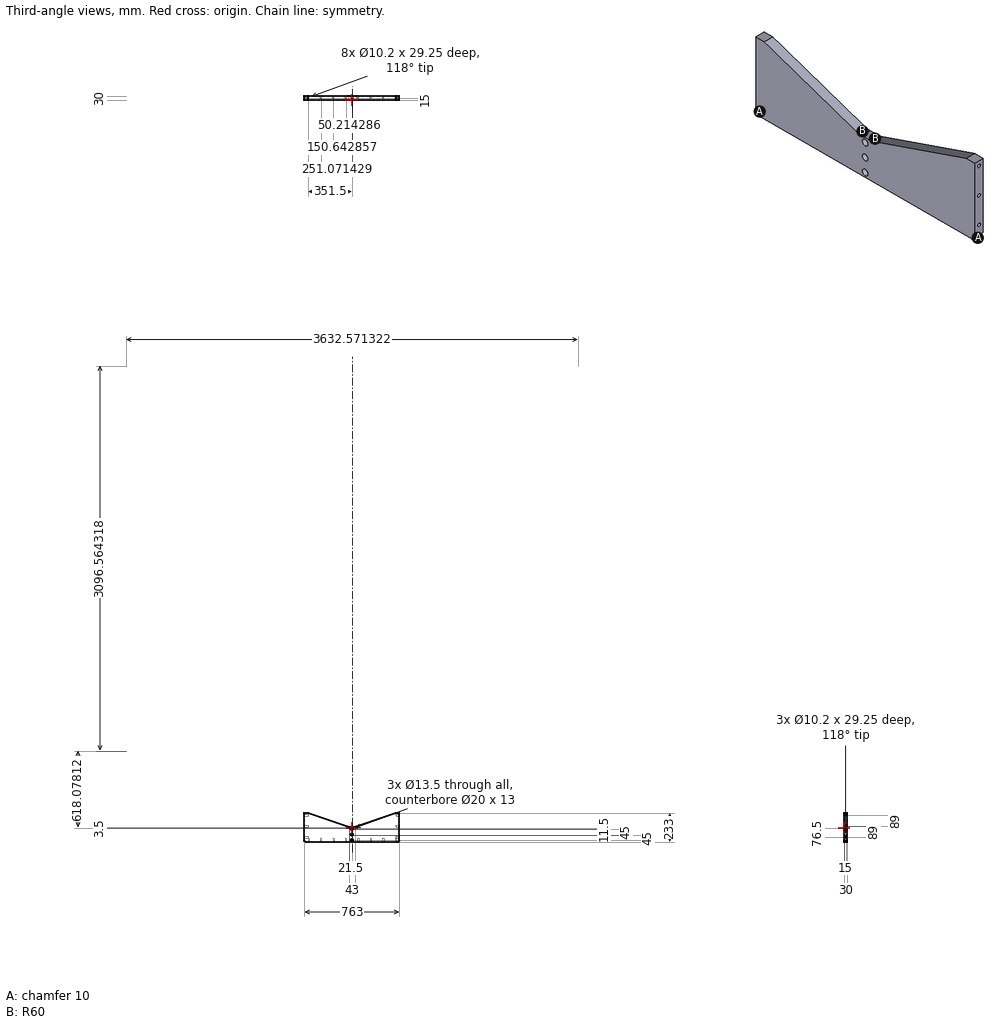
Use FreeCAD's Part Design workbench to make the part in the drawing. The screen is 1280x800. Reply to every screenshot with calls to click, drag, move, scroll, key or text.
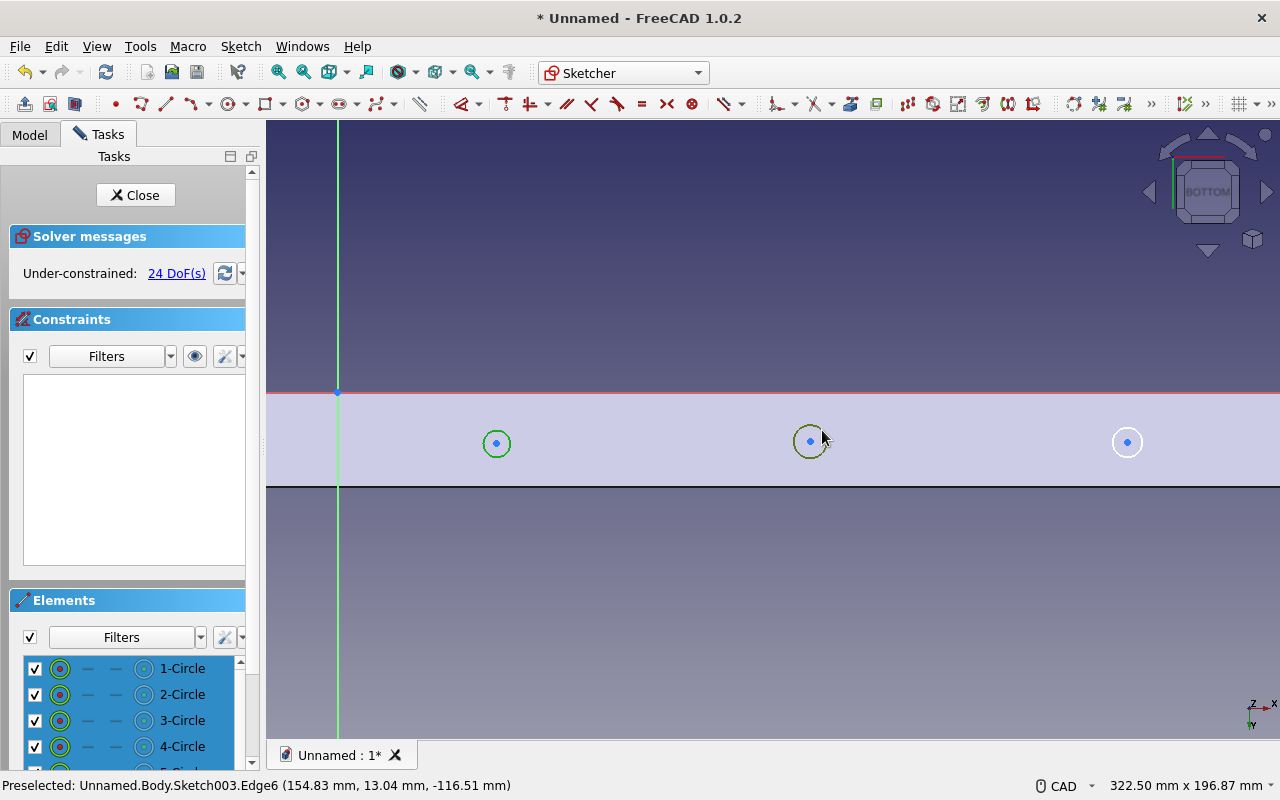
click(1113, 442)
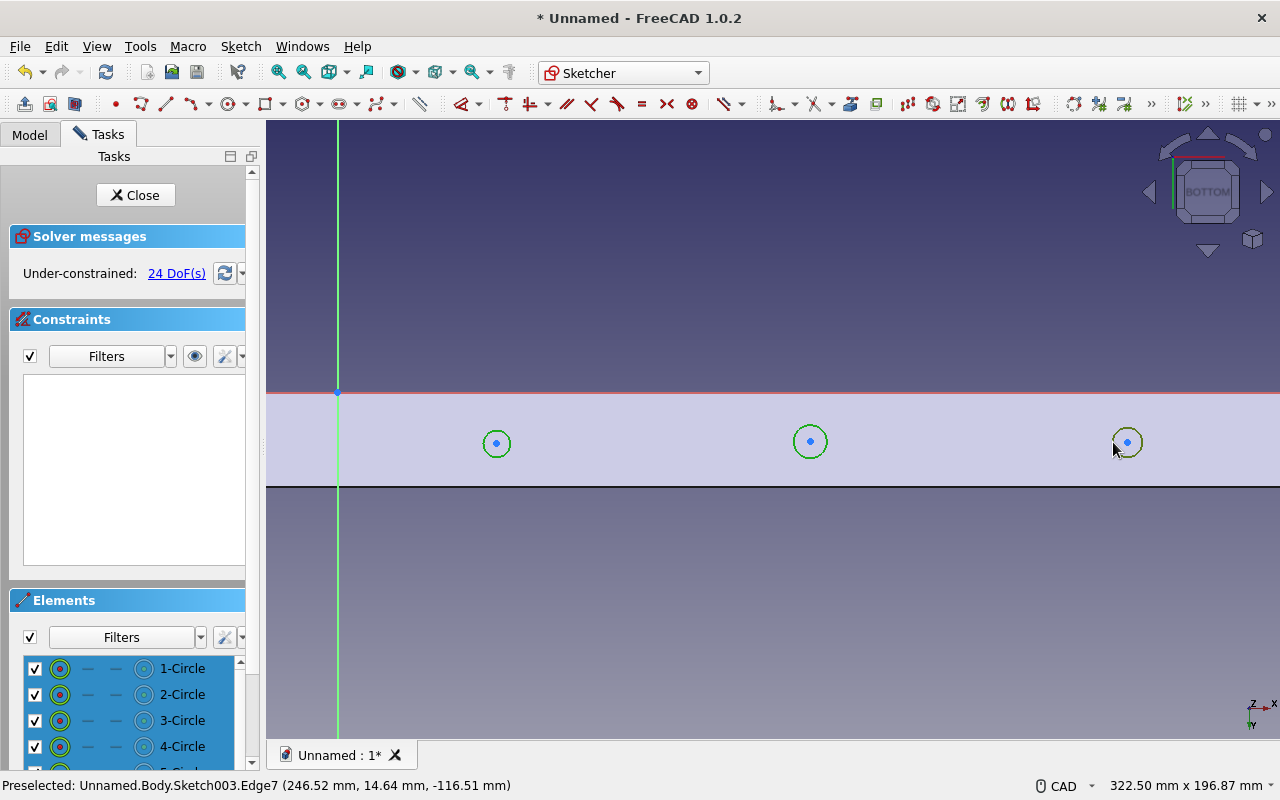
scroll(824, 431, down, 7)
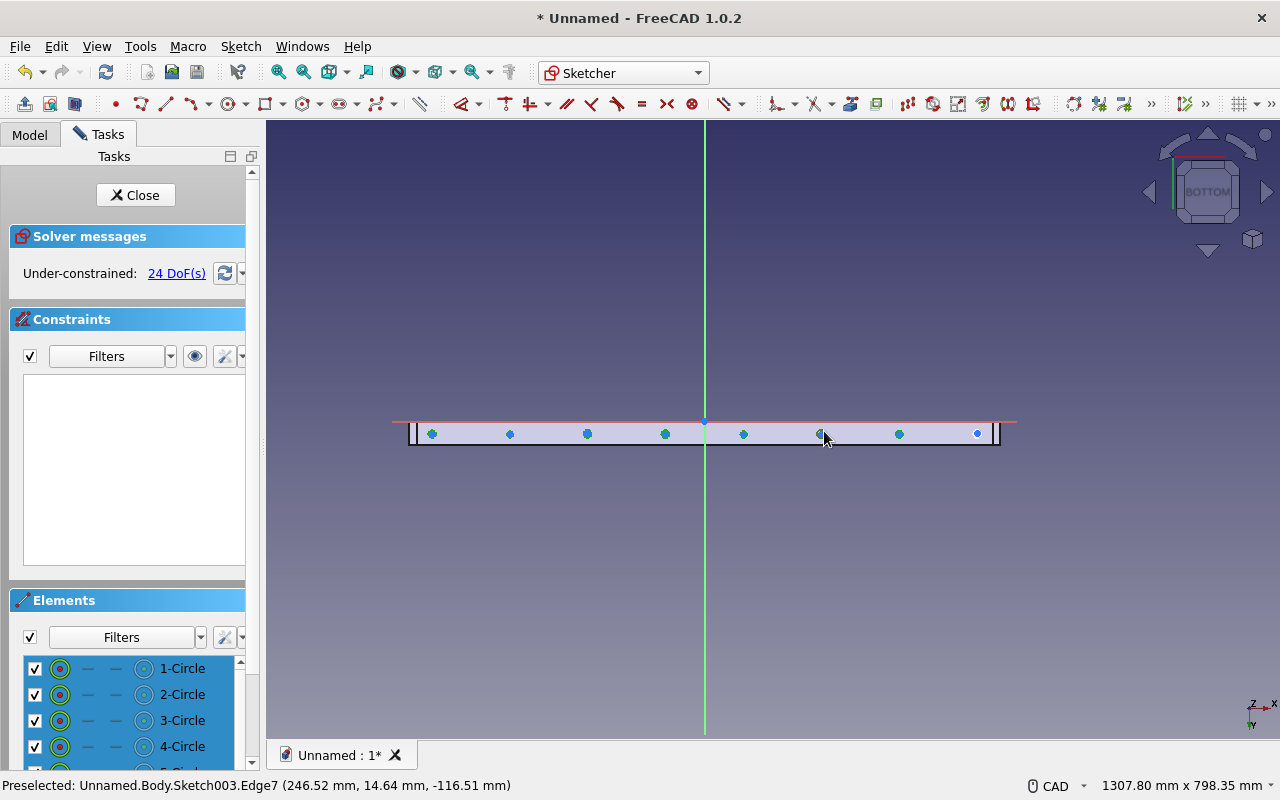
scroll(980, 431, up, 7)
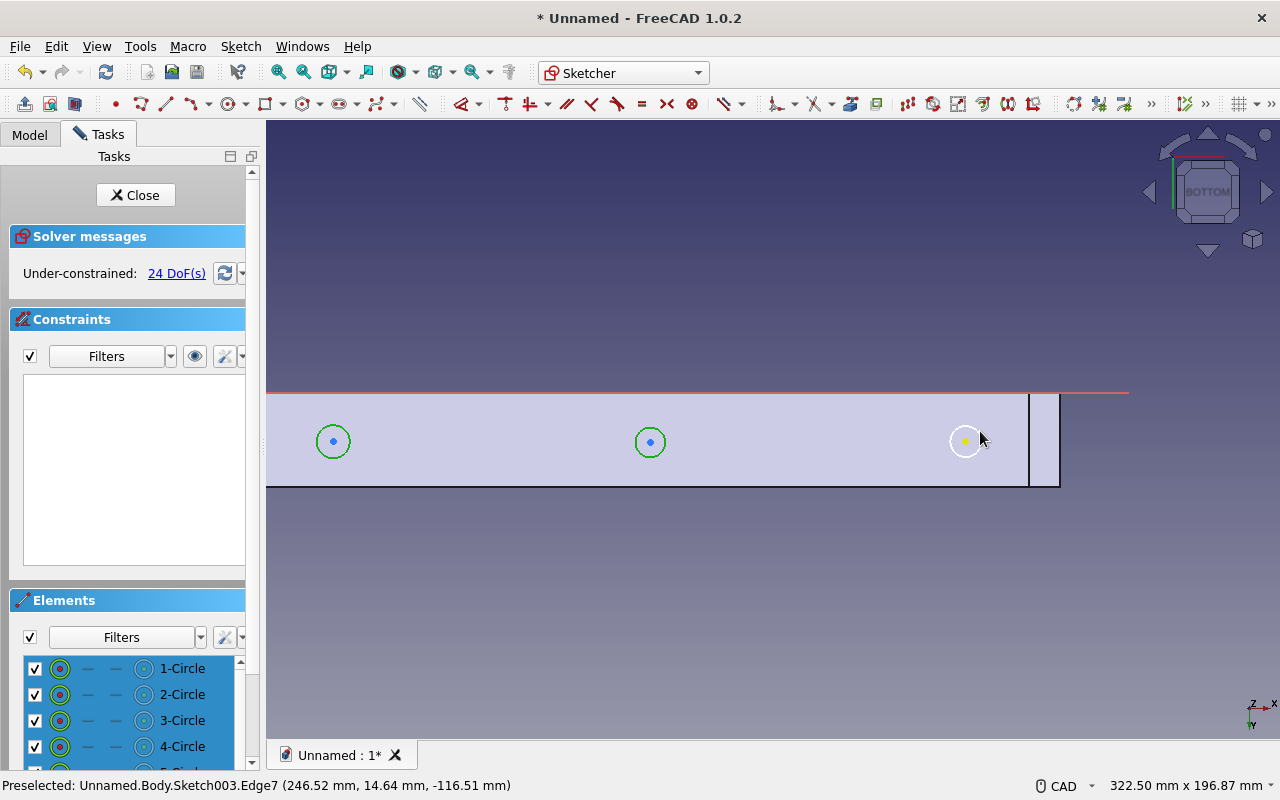
click(977, 431)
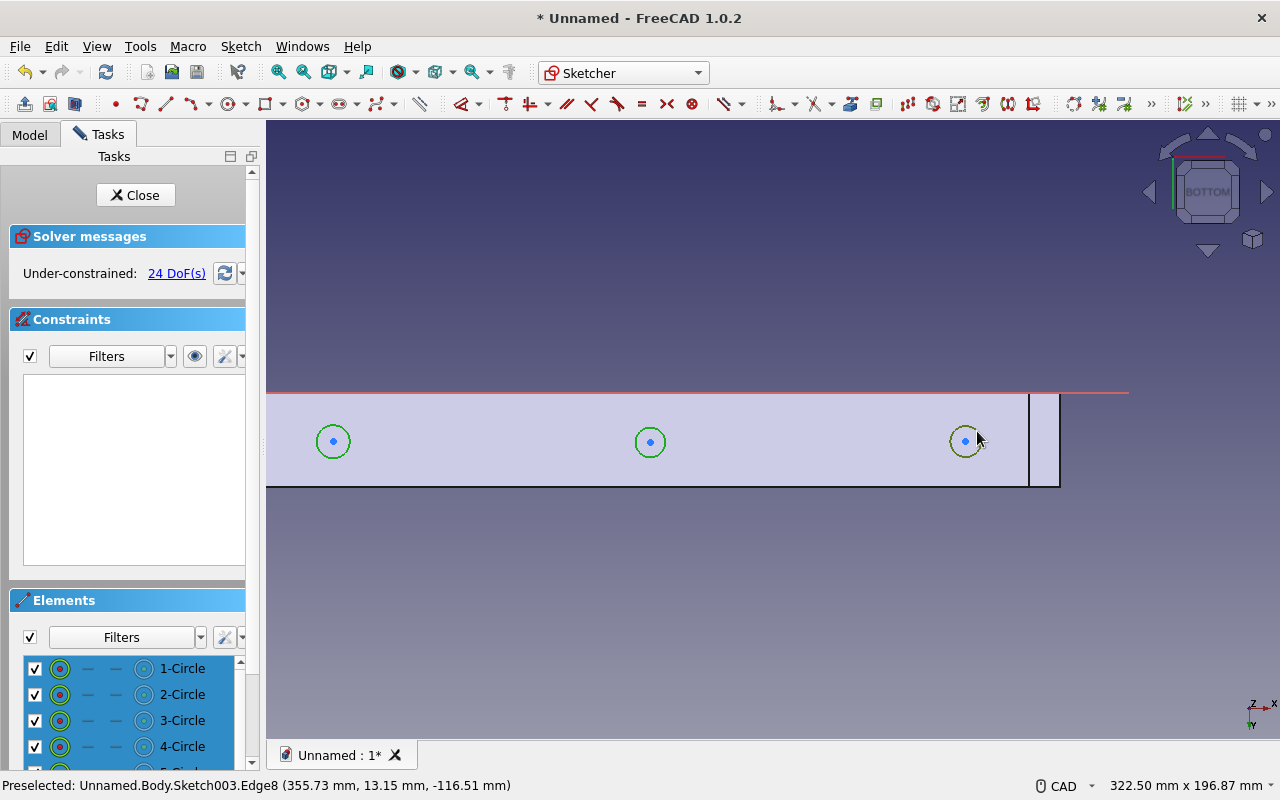
key(e)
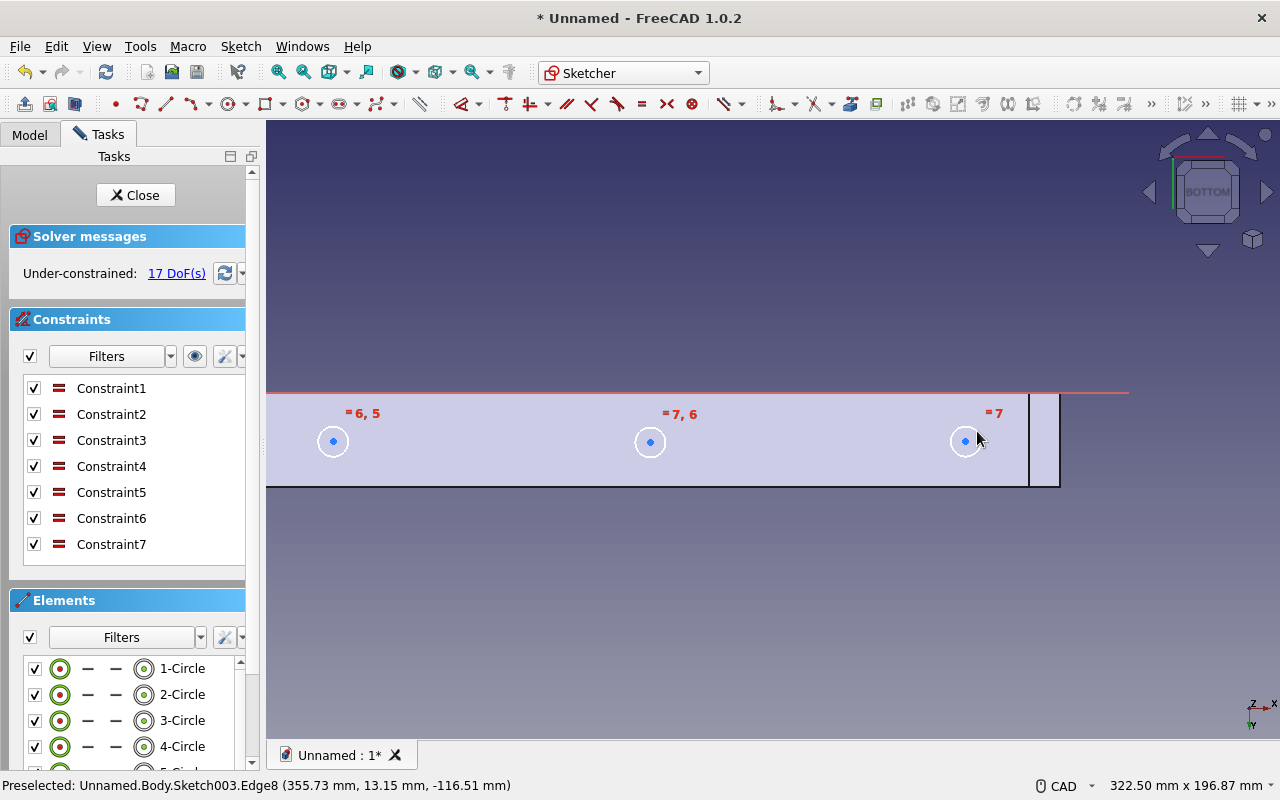
scroll(981, 431, down, 7)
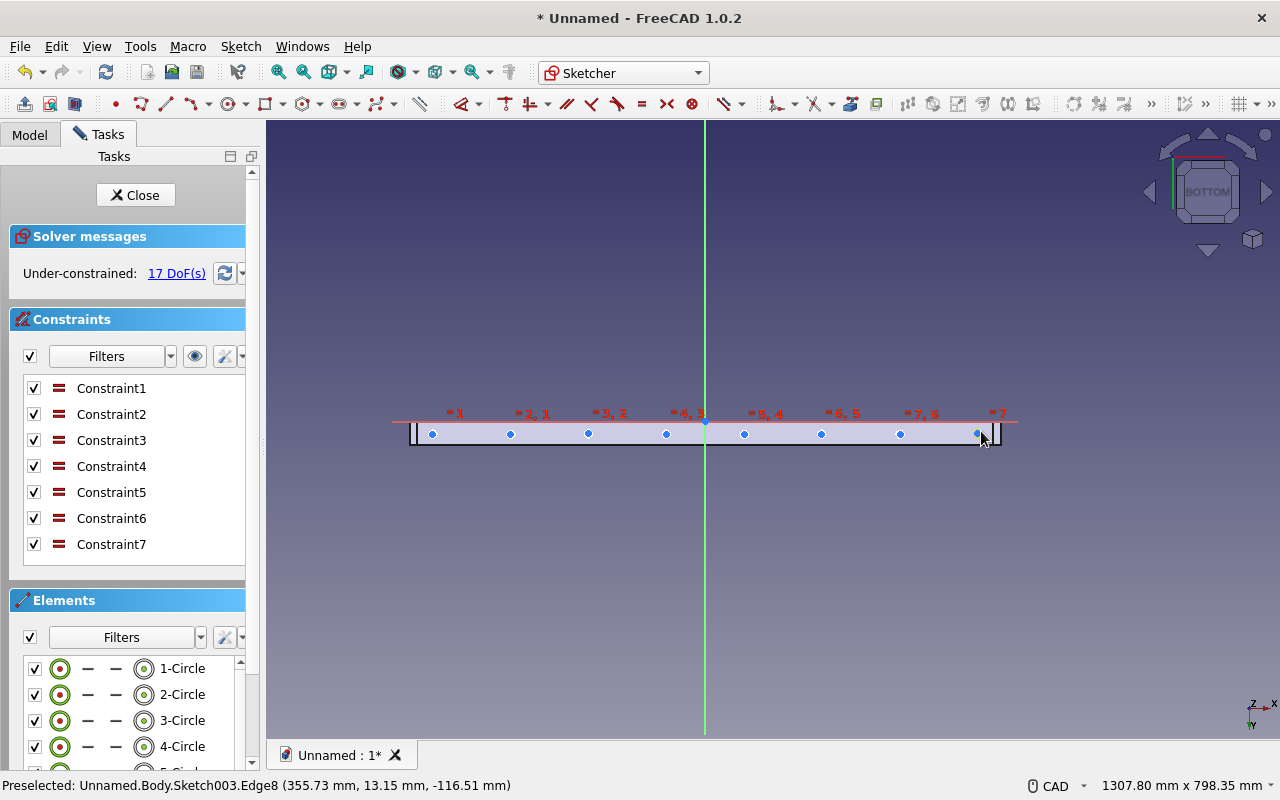
click(666, 434)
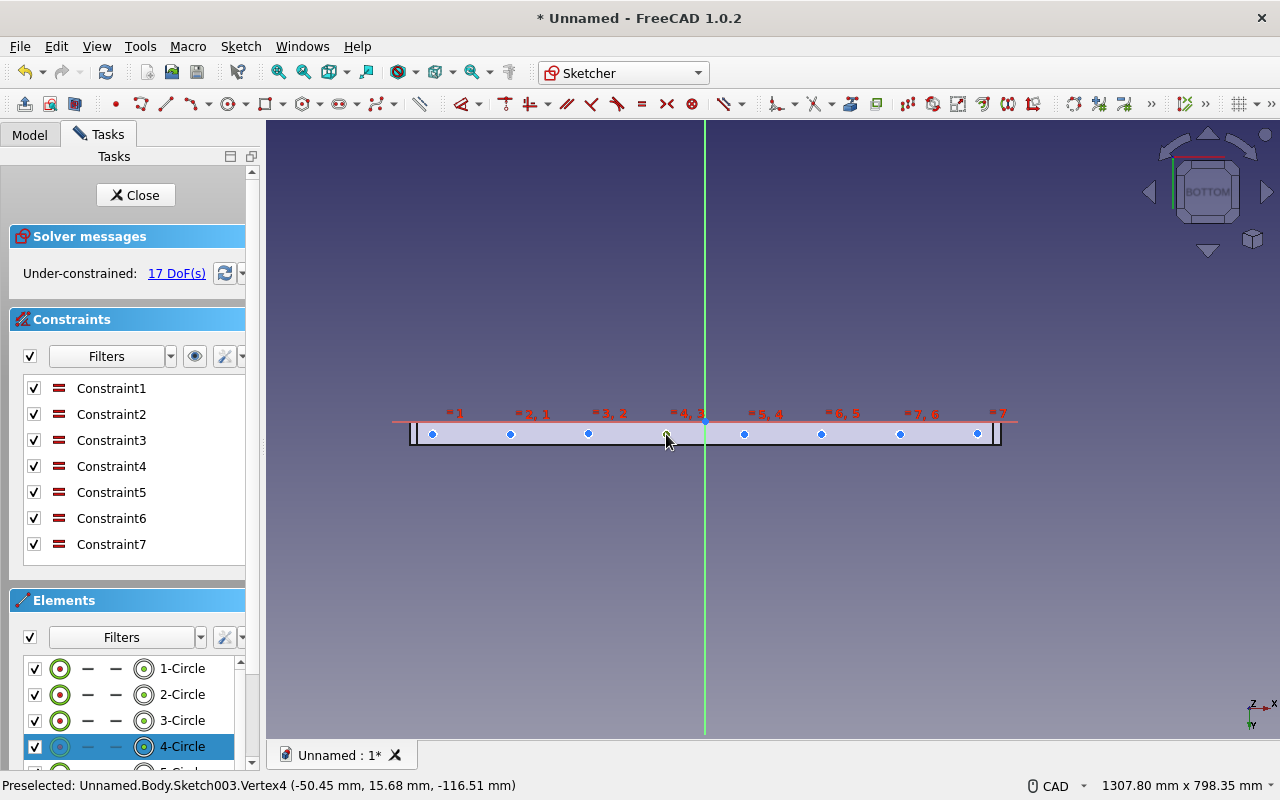
click(744, 435)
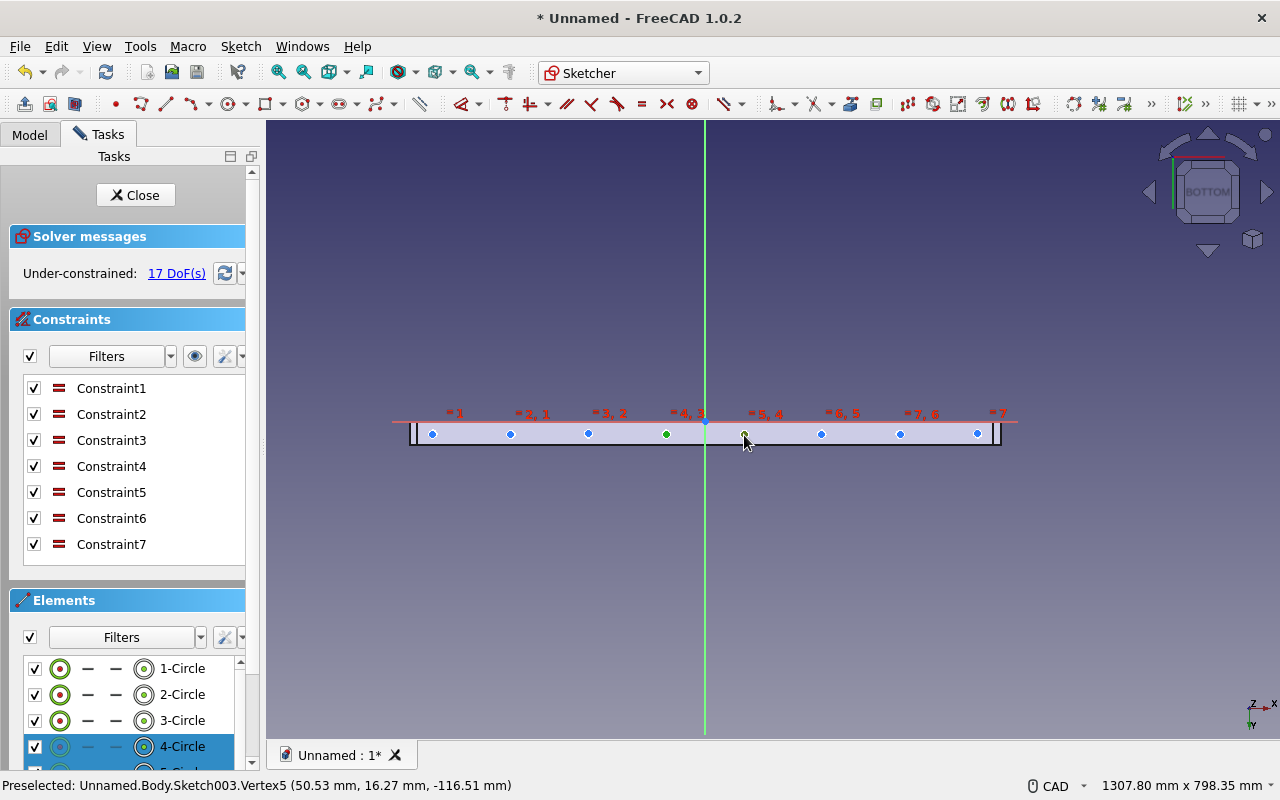
click(705, 671)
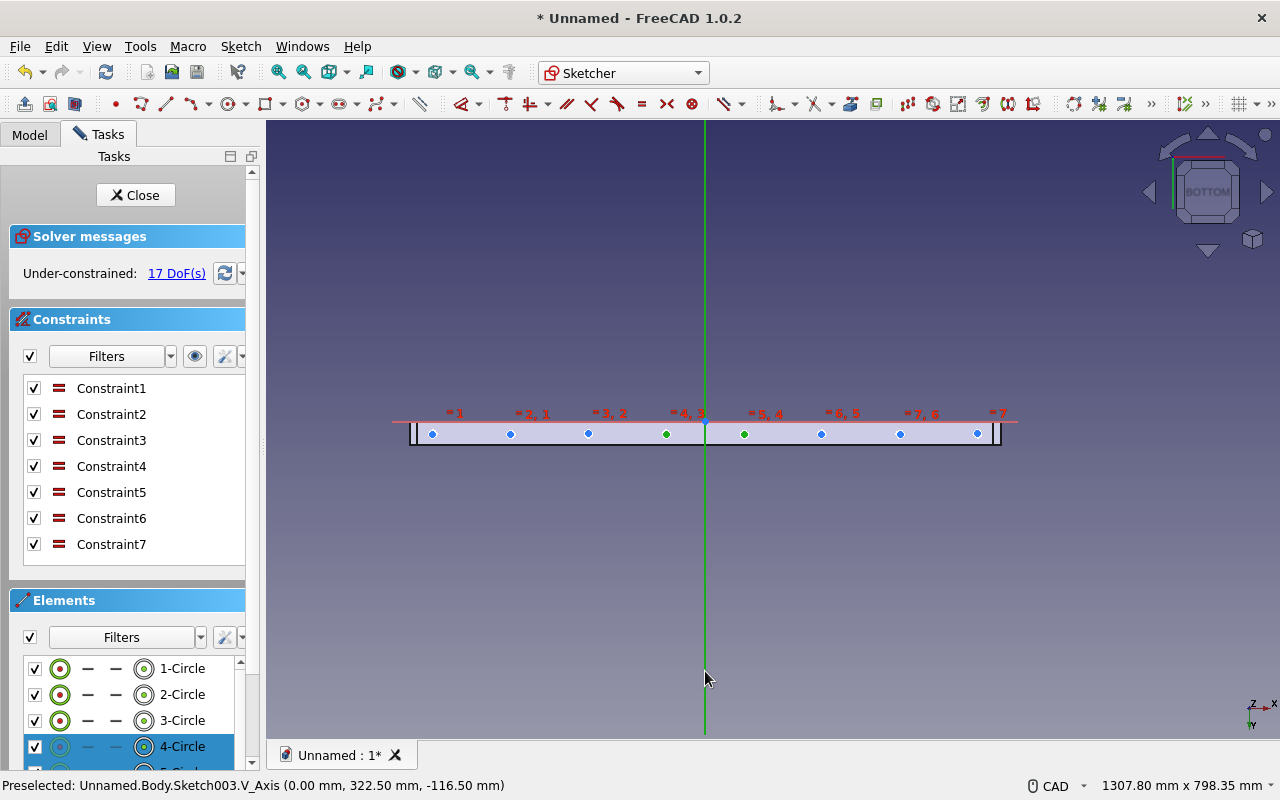
click(667, 104)